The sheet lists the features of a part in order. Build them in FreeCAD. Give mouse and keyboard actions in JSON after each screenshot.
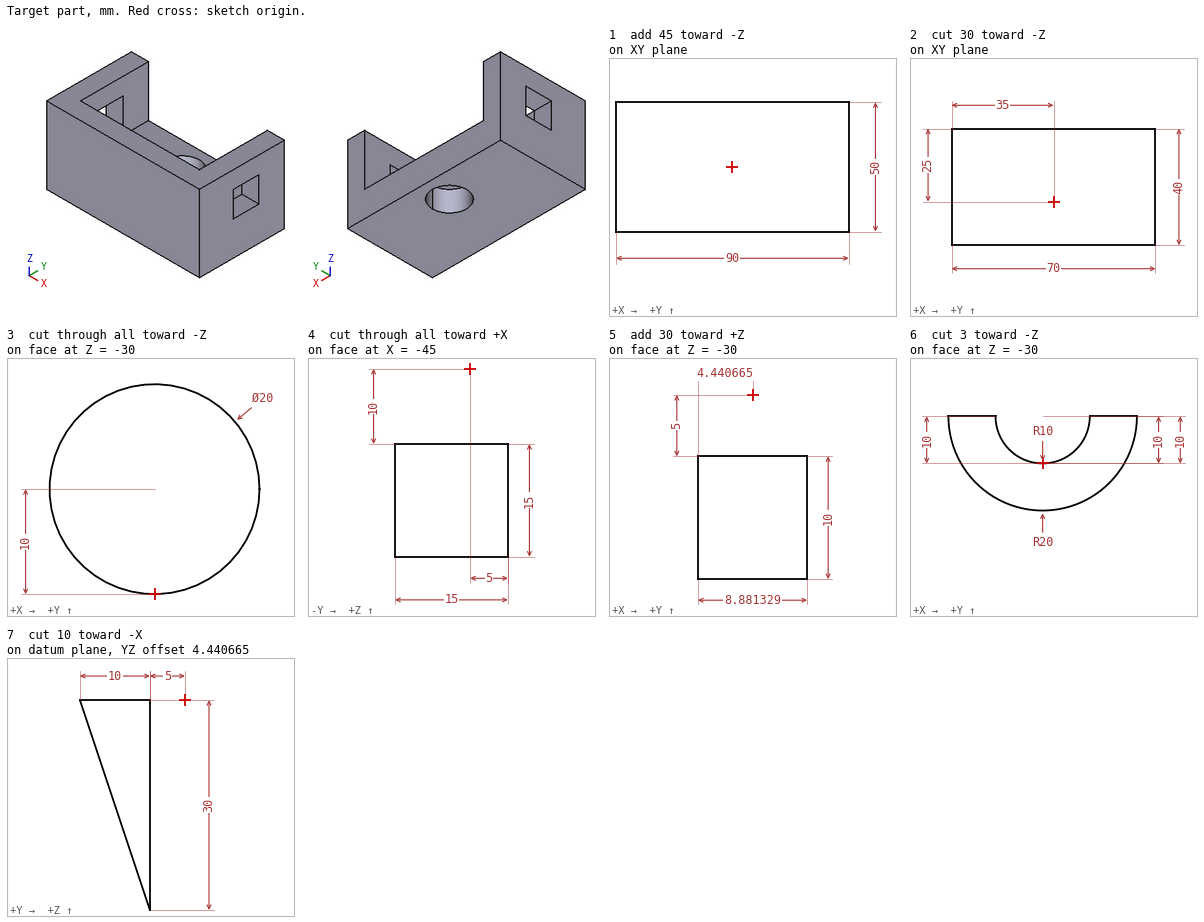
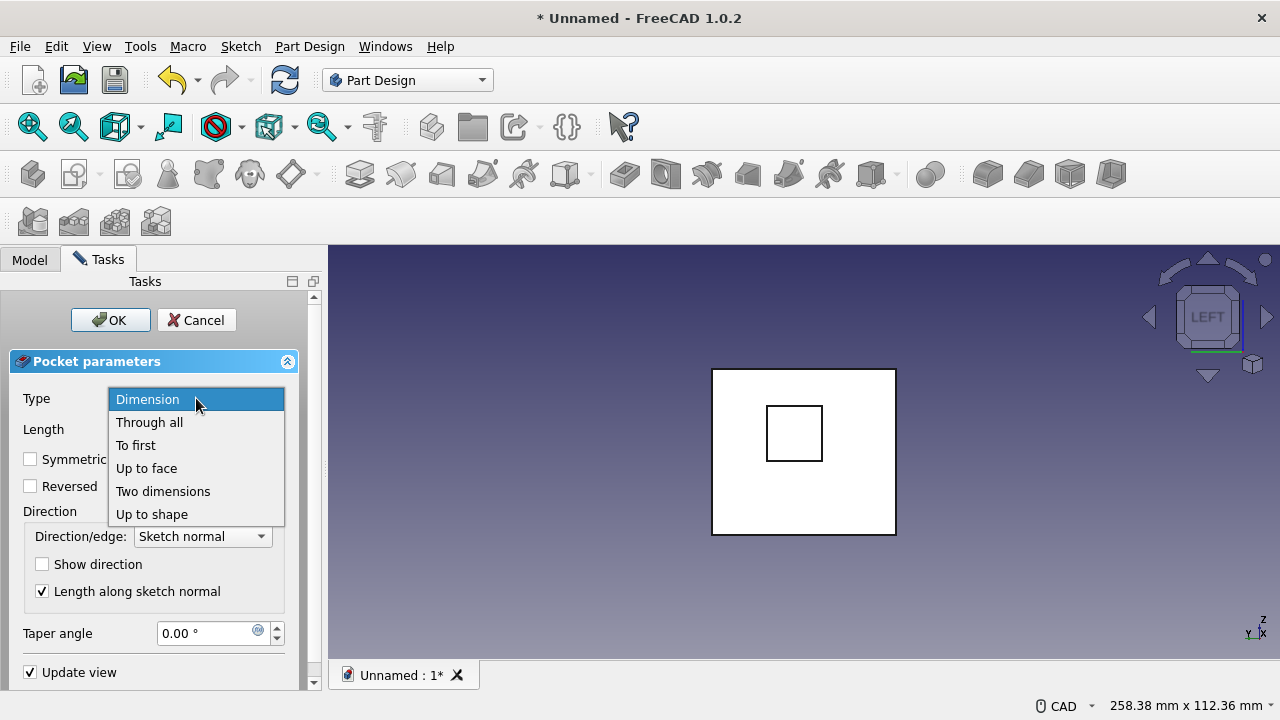
{"action": "left_click", "coordinate": [194, 422]}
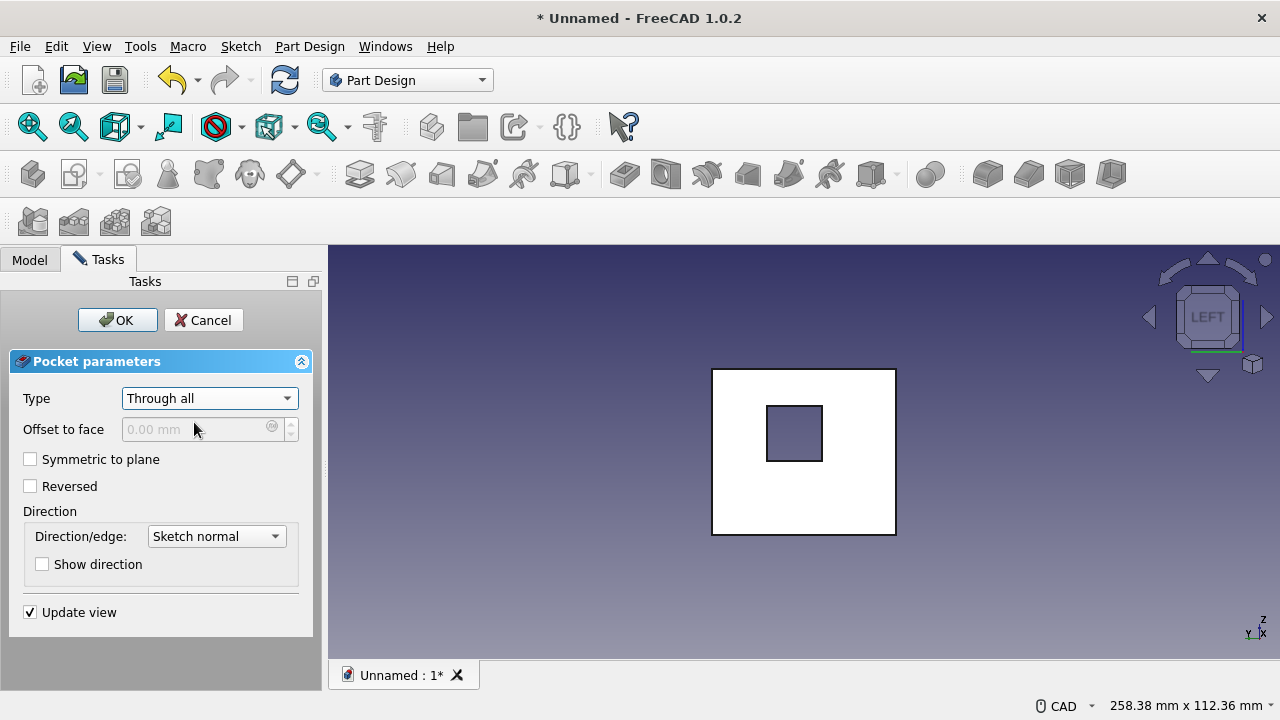
{"action": "left_click", "coordinate": [118, 320]}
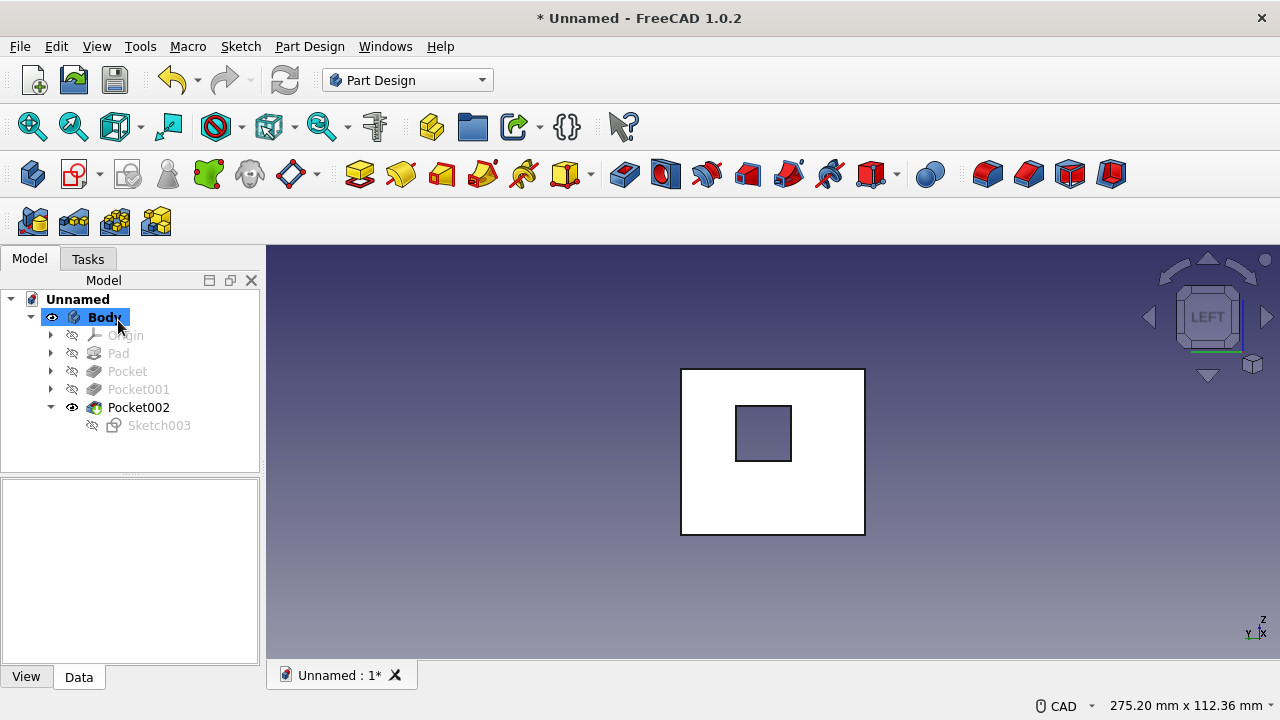
{"action": "key", "text": "v f"}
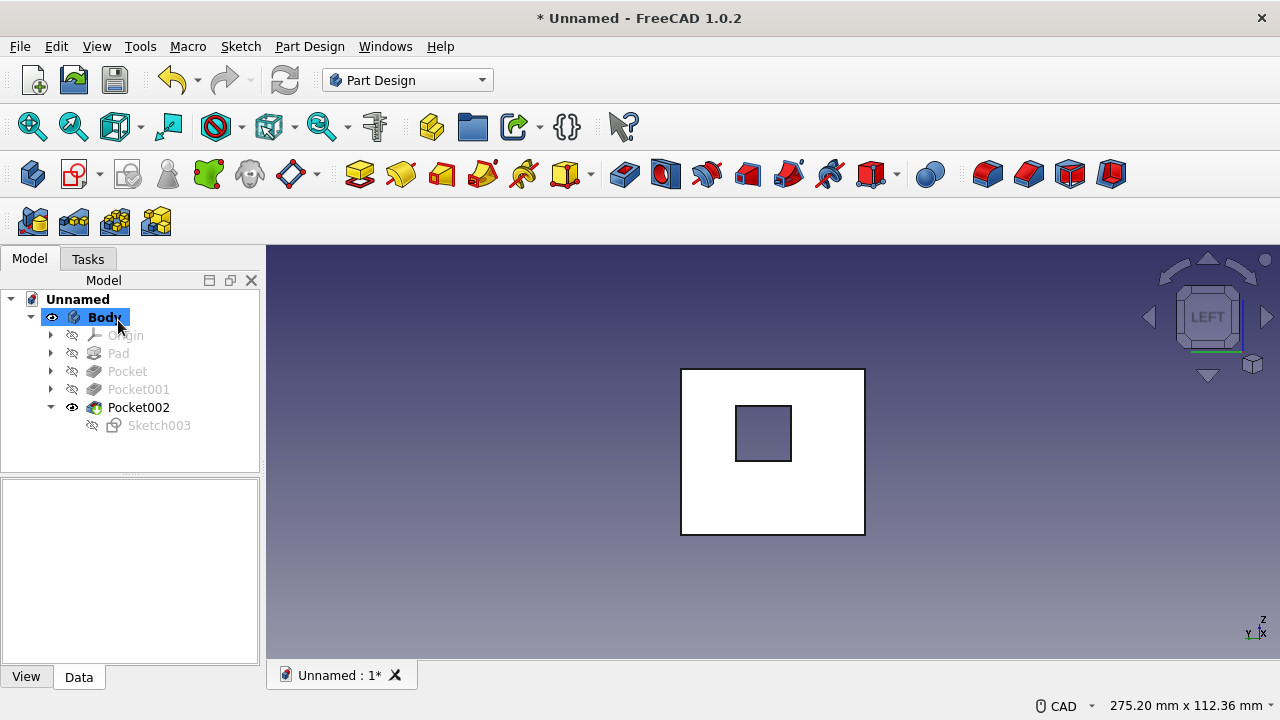
{"action": "key", "text": "0"}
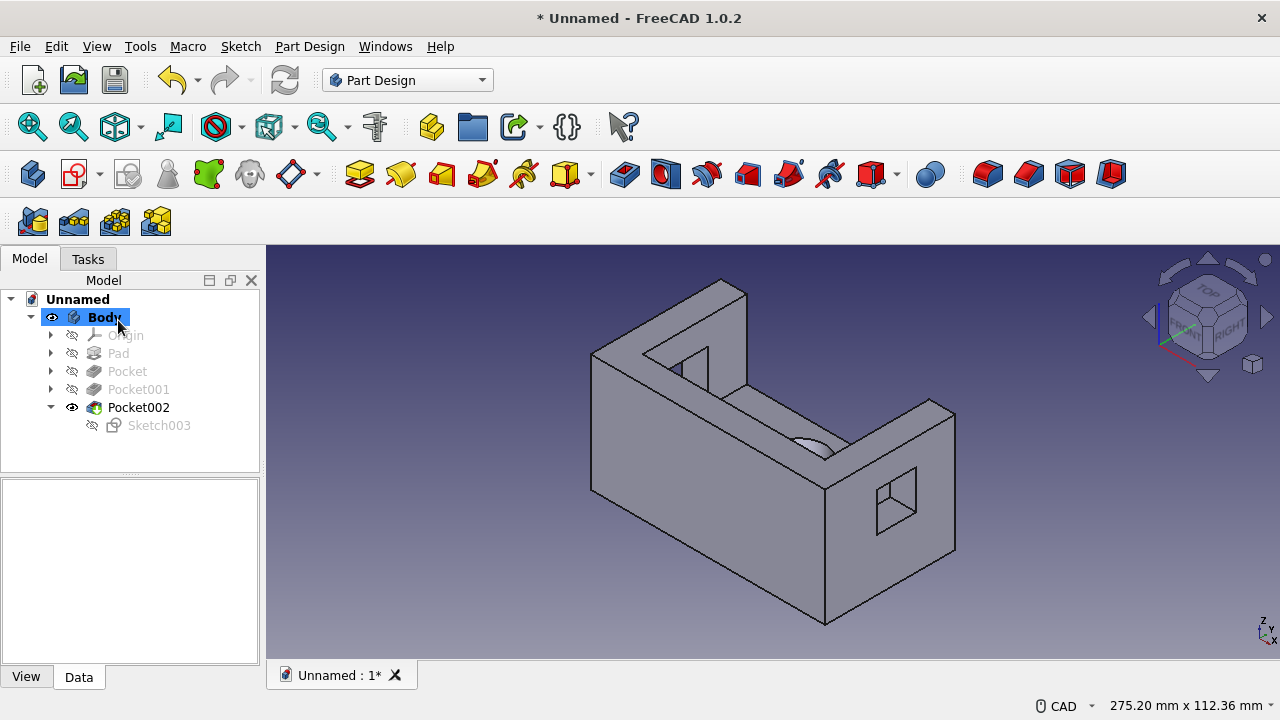
{"action": "key", "text": "2"}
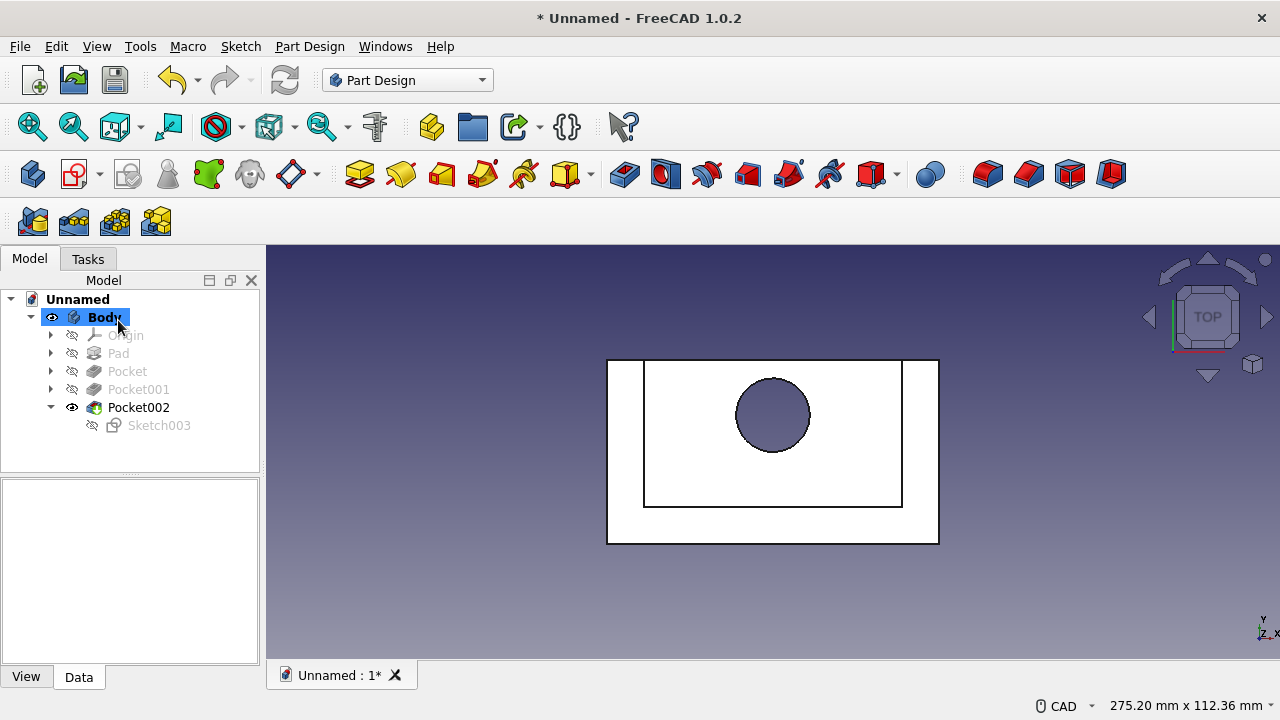
{"action": "key", "text": "v f"}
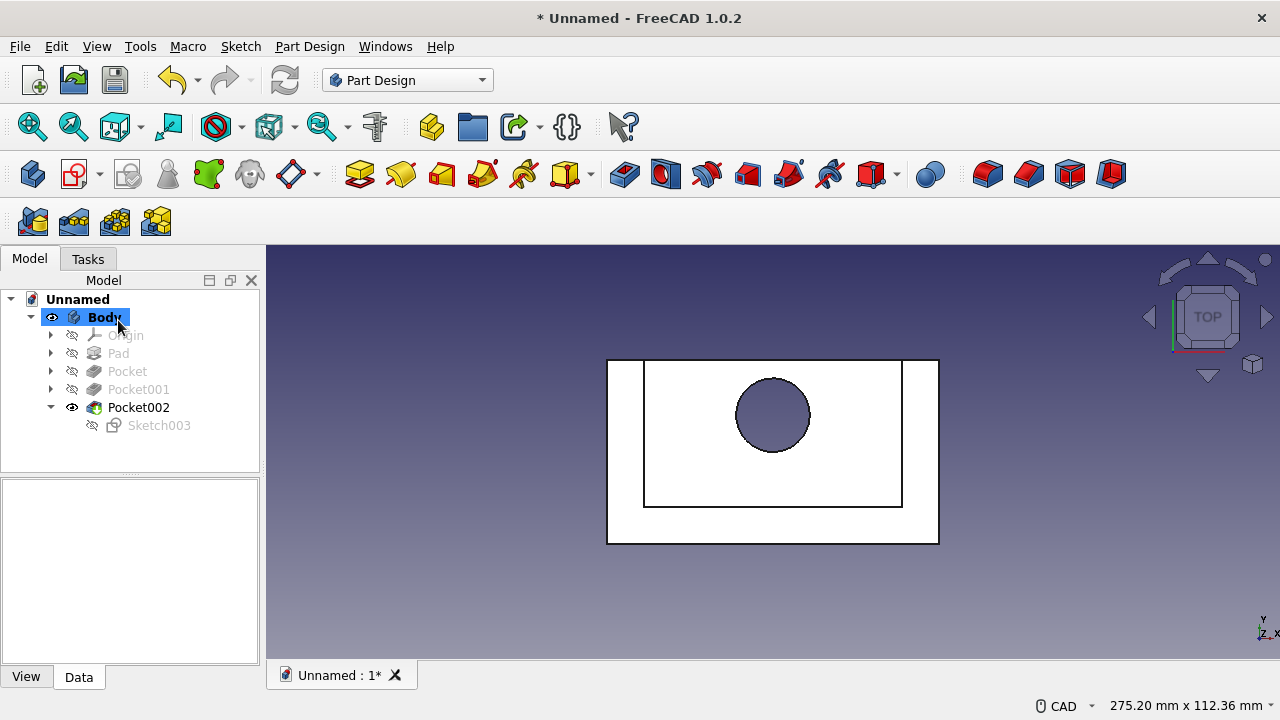
{"action": "left_click", "coordinate": [847, 454]}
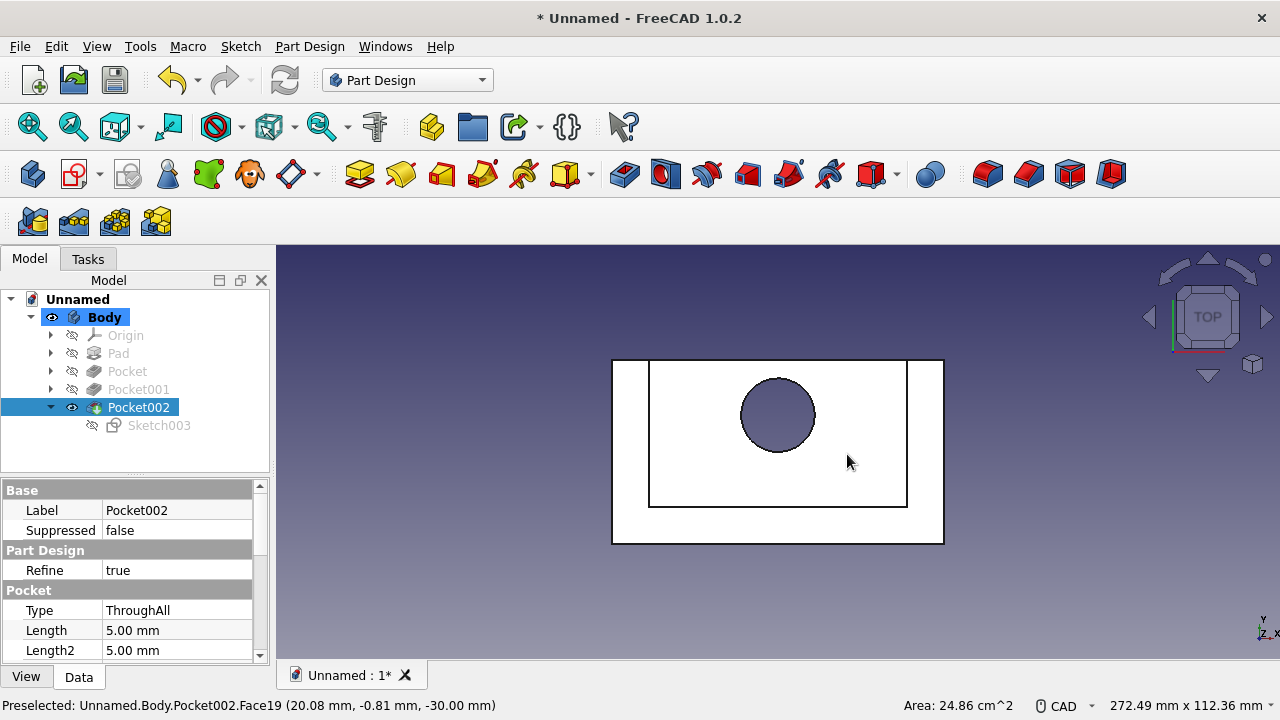
{"action": "left_click", "coordinate": [74, 174]}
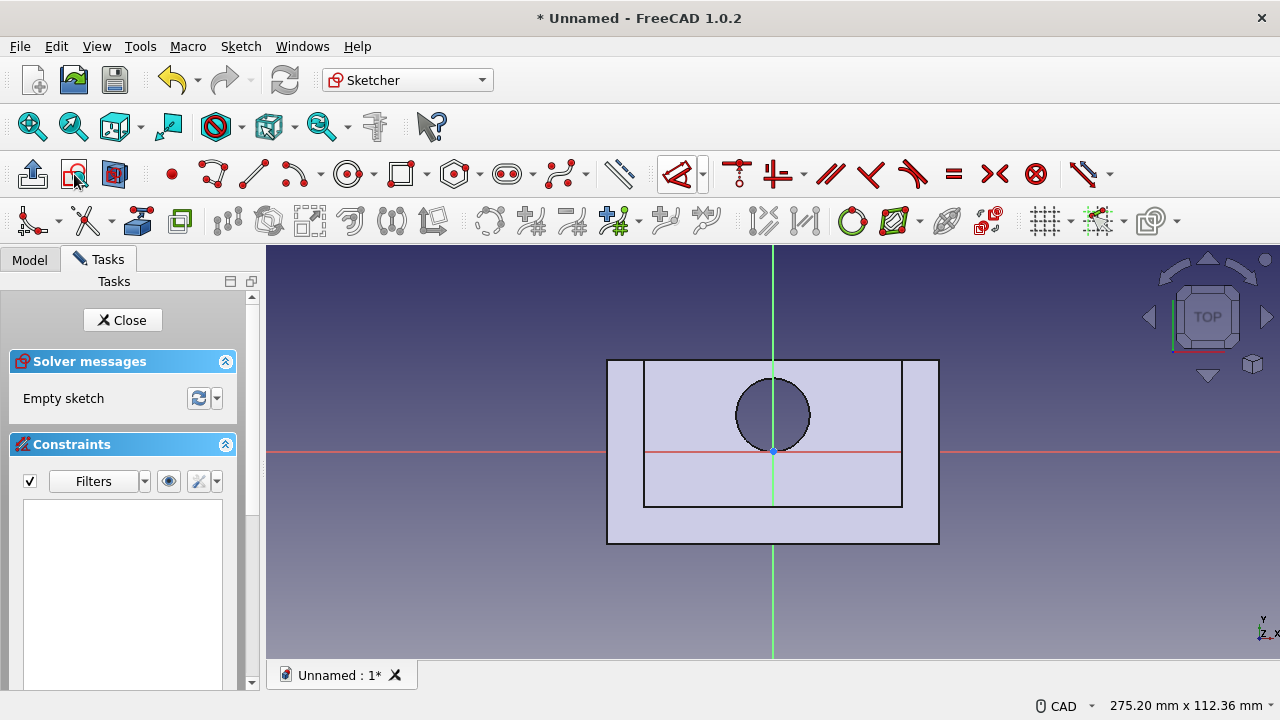
{"action": "scroll", "coordinate": [790, 487], "scroll_direction": "up", "scroll_amount": 8}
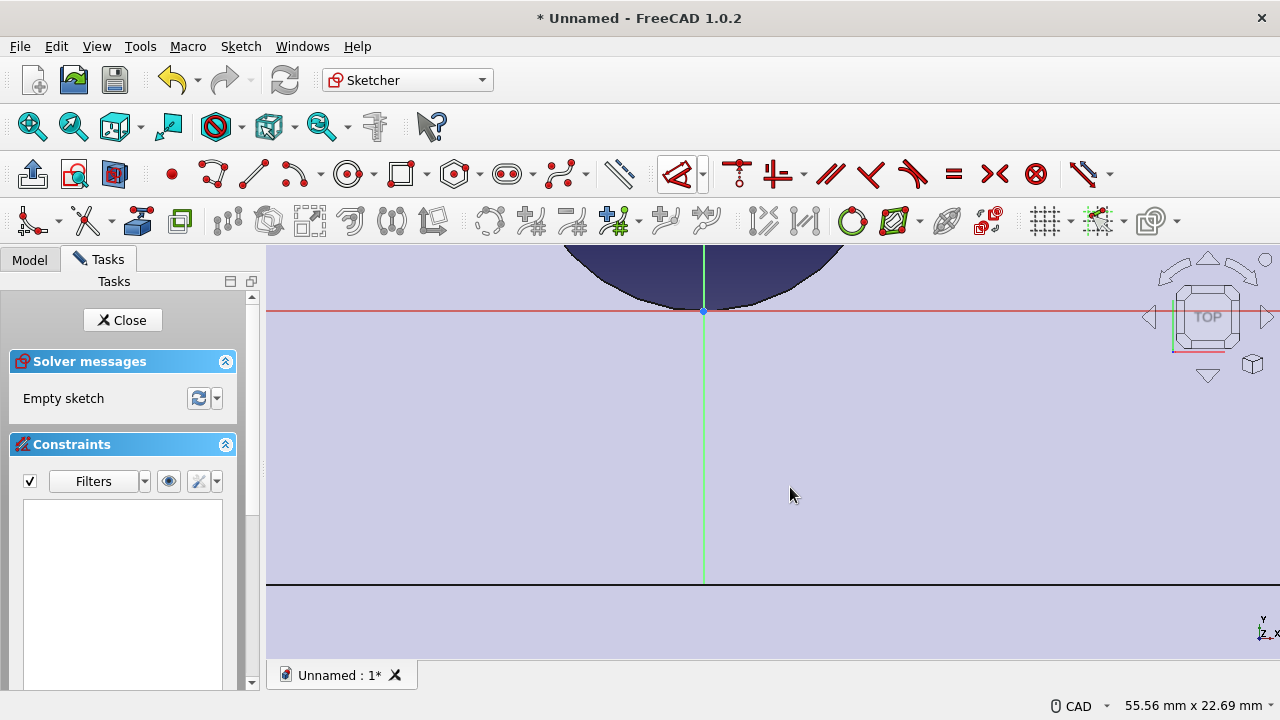
{"action": "key", "text": "g r"}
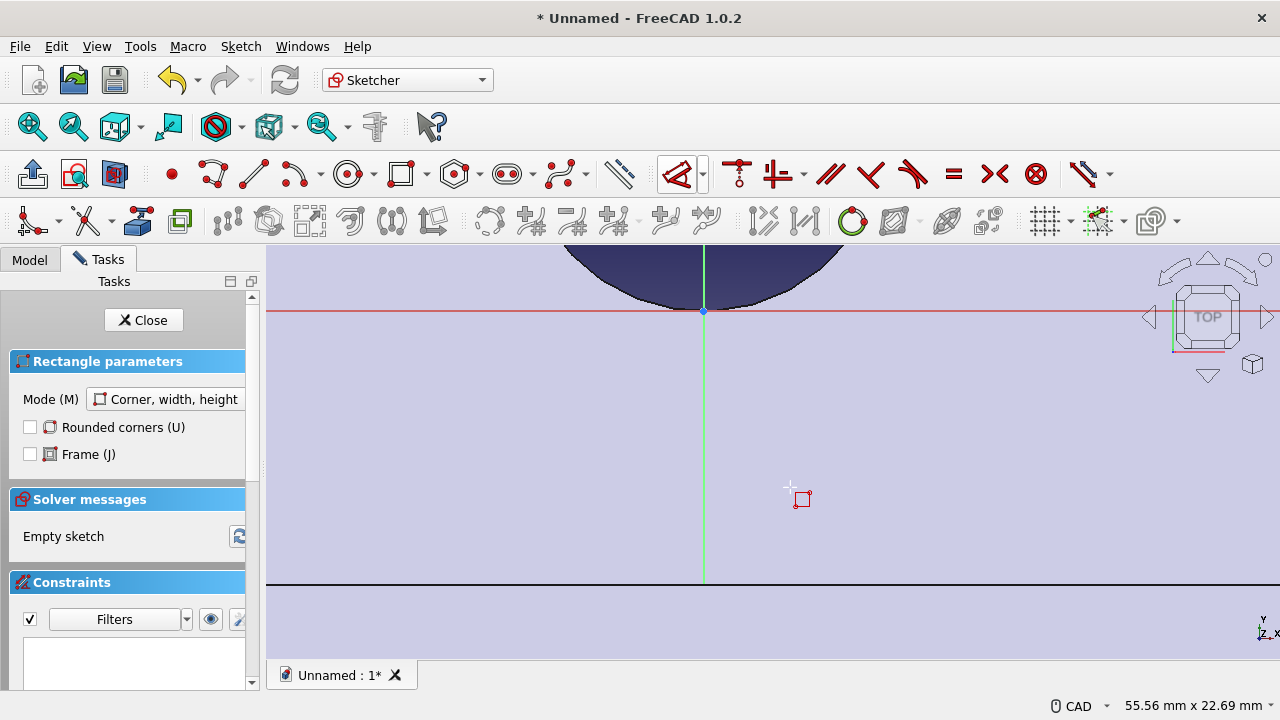
{"action": "left_click", "coordinate": [623, 403]}
{"action": "mouse_move", "coordinate": [785, 585]}